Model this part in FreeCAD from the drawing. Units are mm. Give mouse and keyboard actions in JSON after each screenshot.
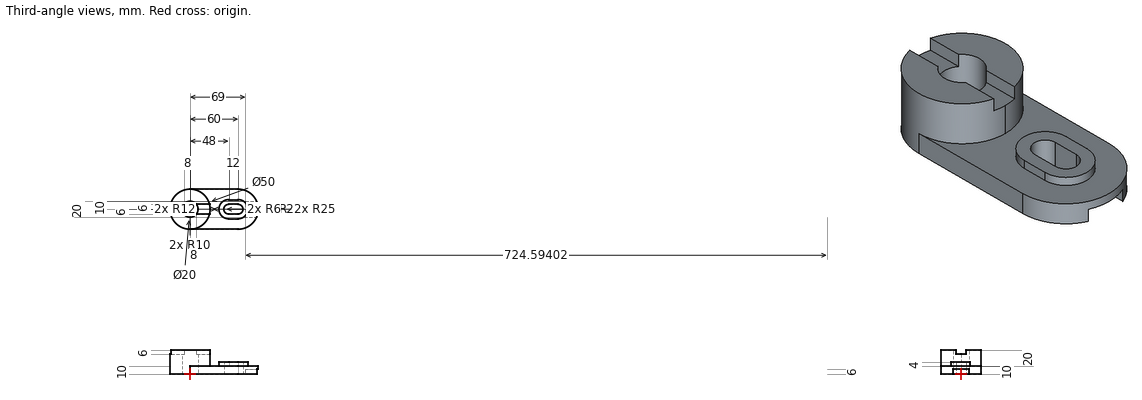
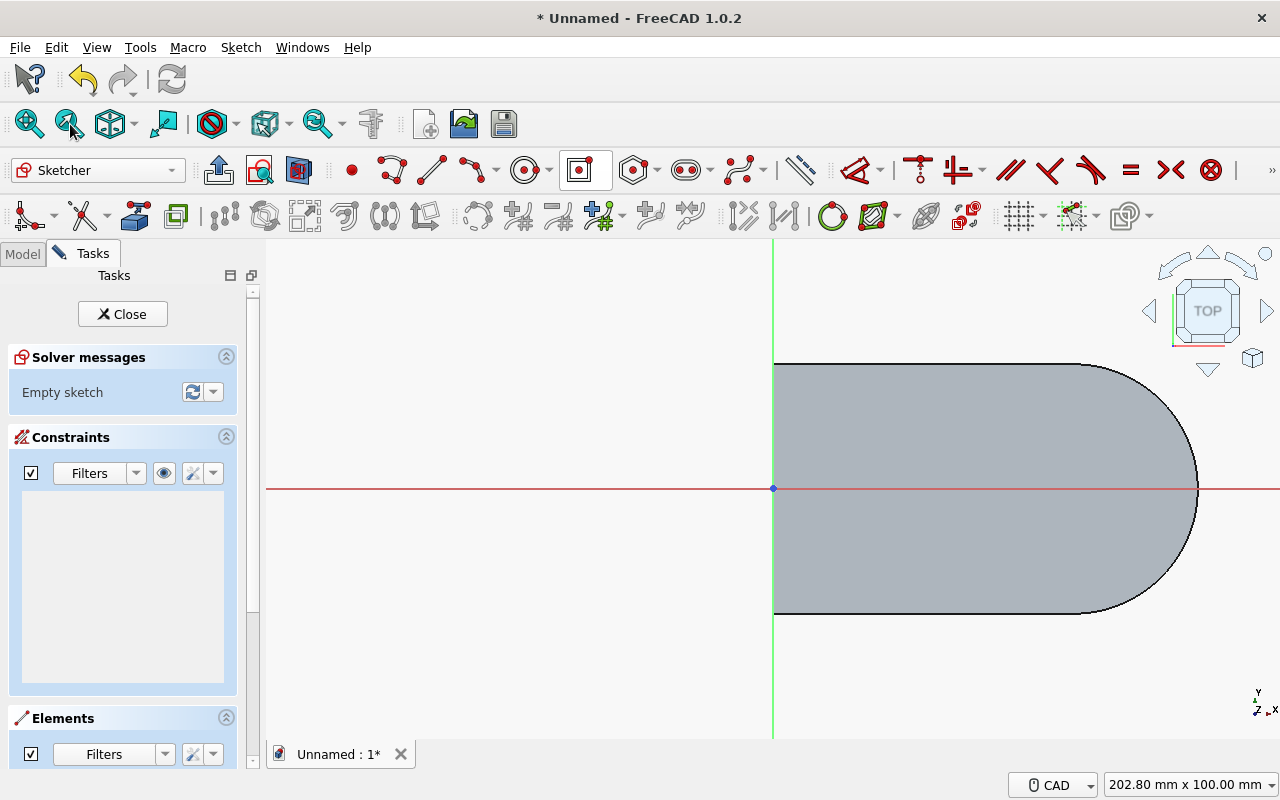
{"action": "left_click", "coordinate": [526, 170]}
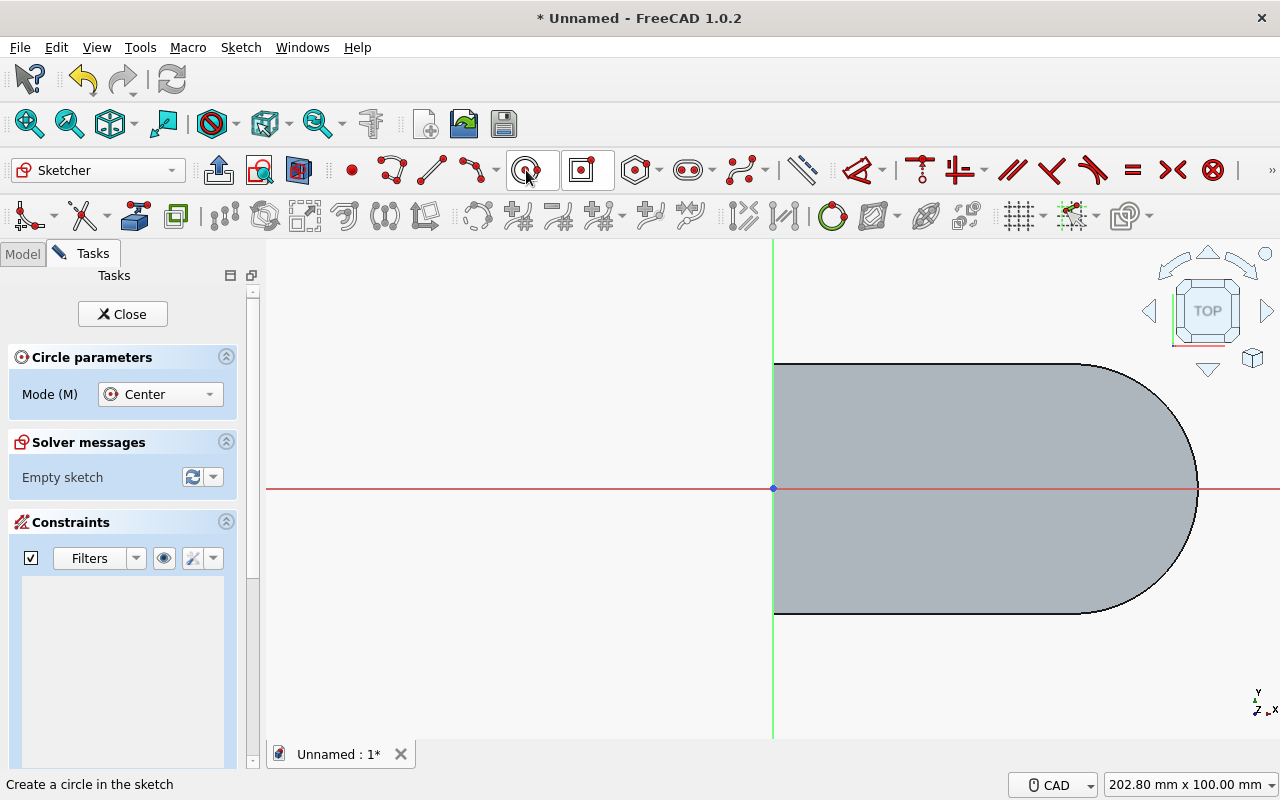
{"action": "left_click", "coordinate": [773, 489]}
{"action": "left_click", "coordinate": [861, 401]}
{"action": "key", "text": "Escape"}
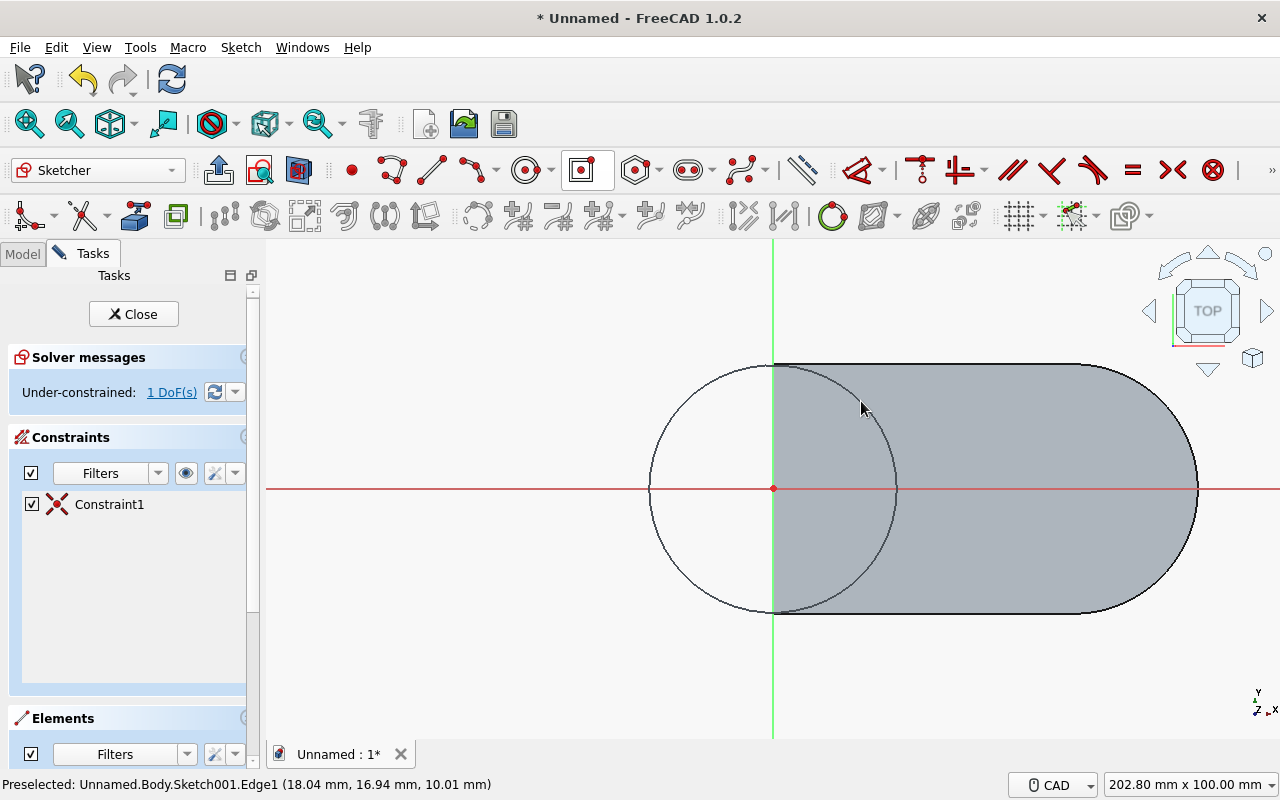
{"action": "left_click", "coordinate": [858, 170]}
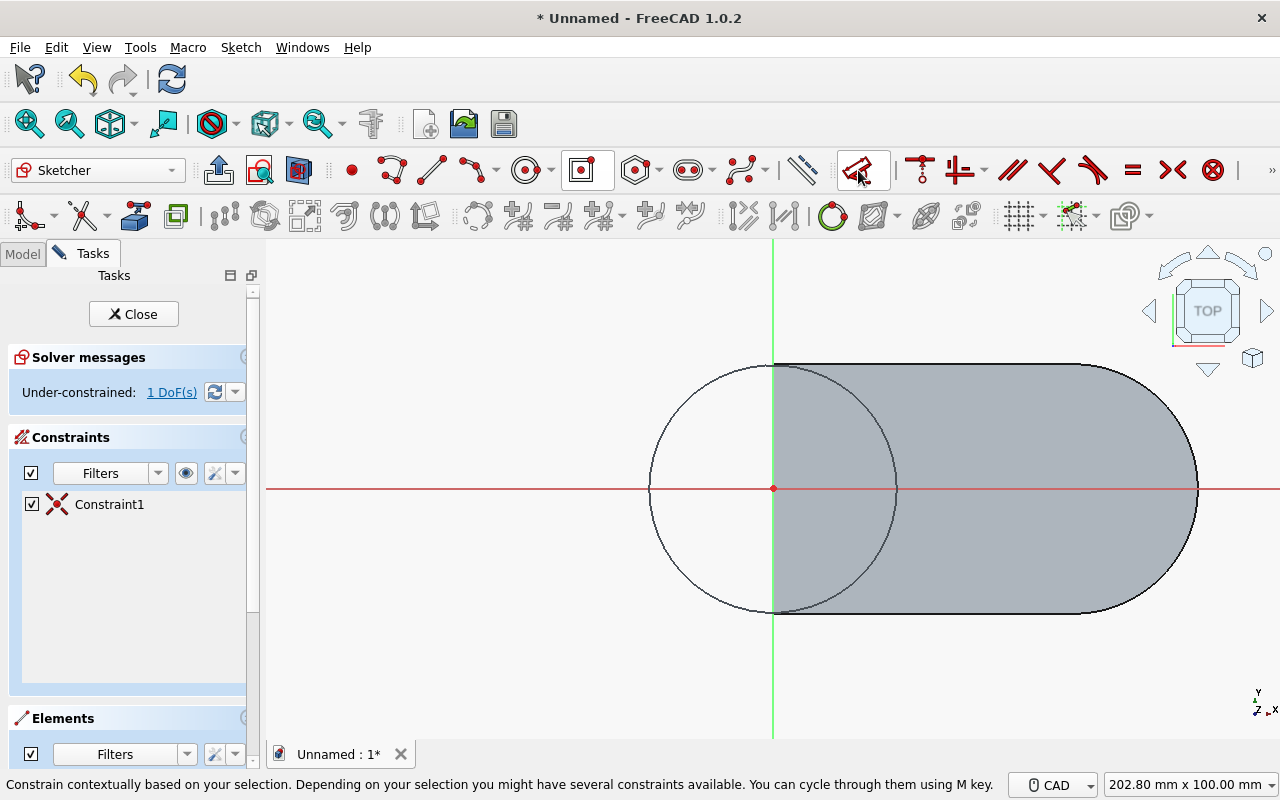
{"action": "left_click", "coordinate": [860, 401]}
{"action": "left_click", "coordinate": [882, 378]}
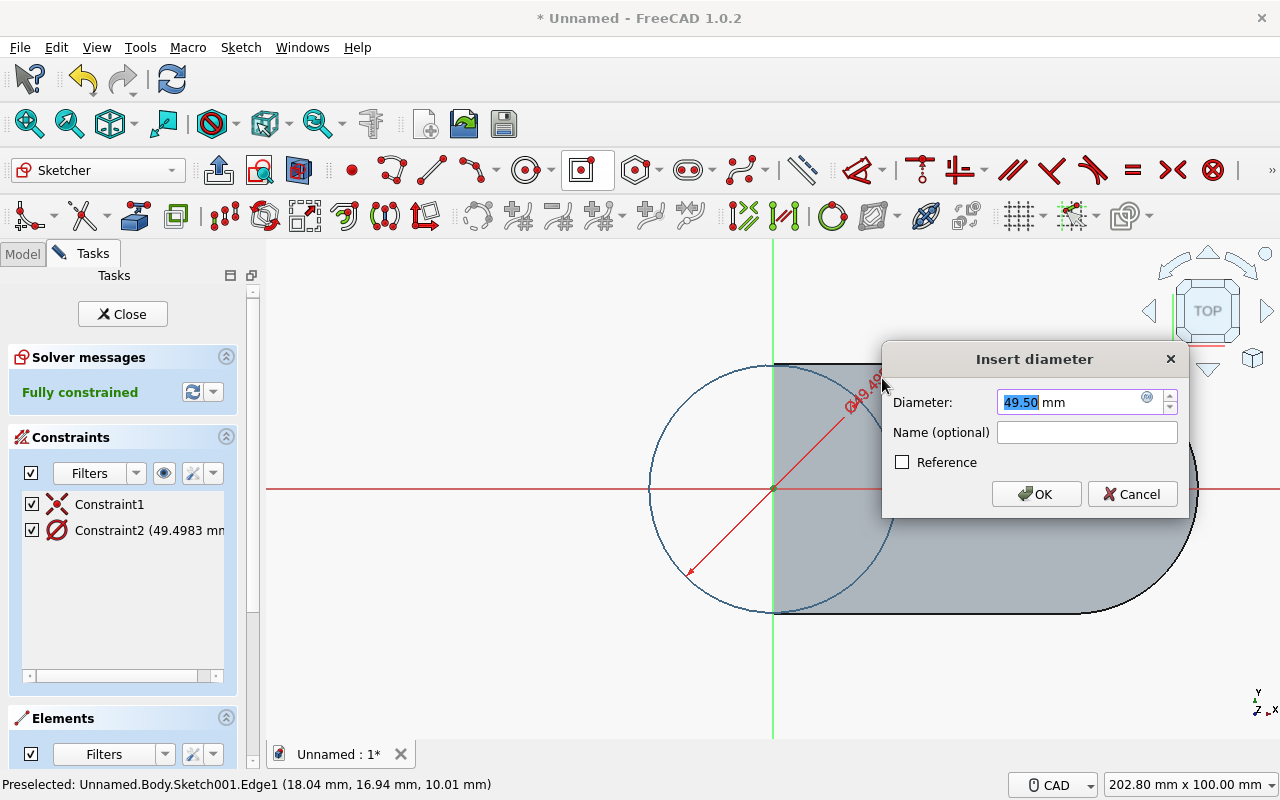
{"action": "type", "text": "50"}
{"action": "key", "text": "Return"}
{"action": "key", "text": "Escape"}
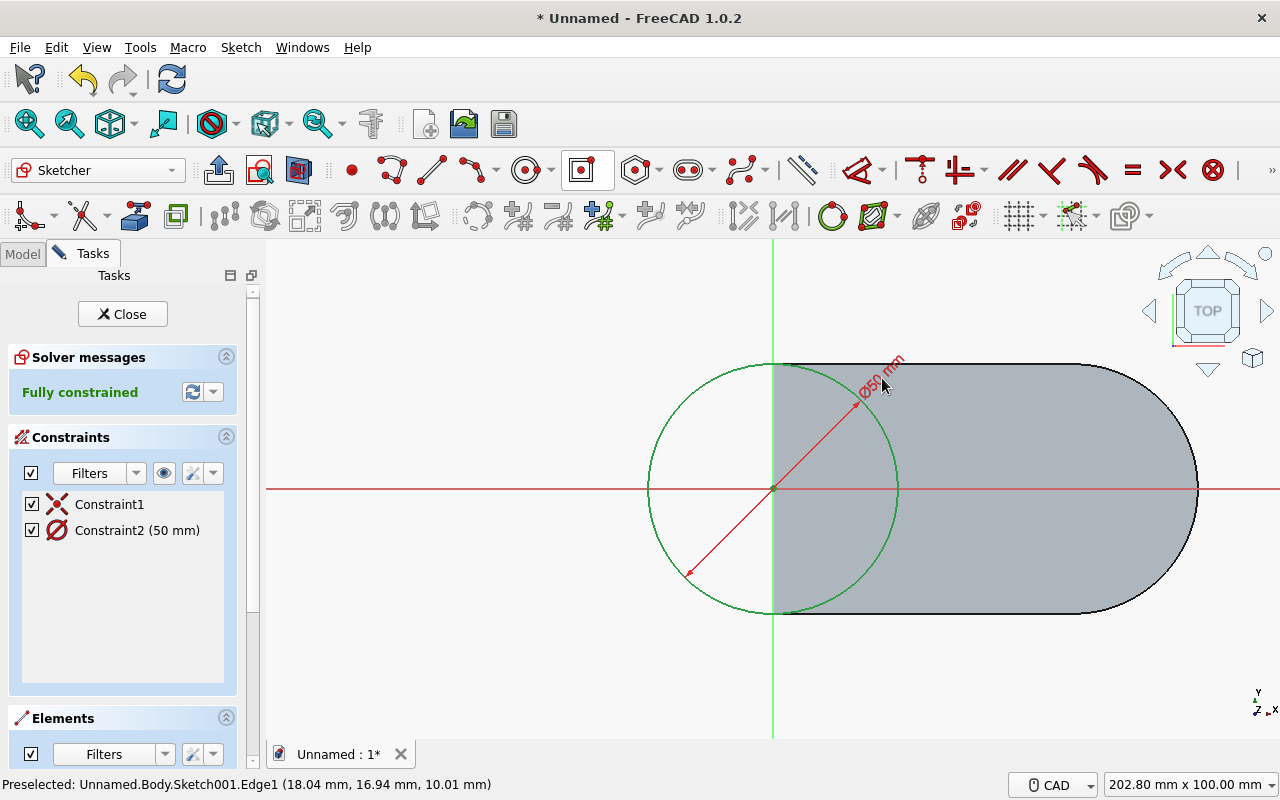
{"action": "left_click", "coordinate": [123, 314]}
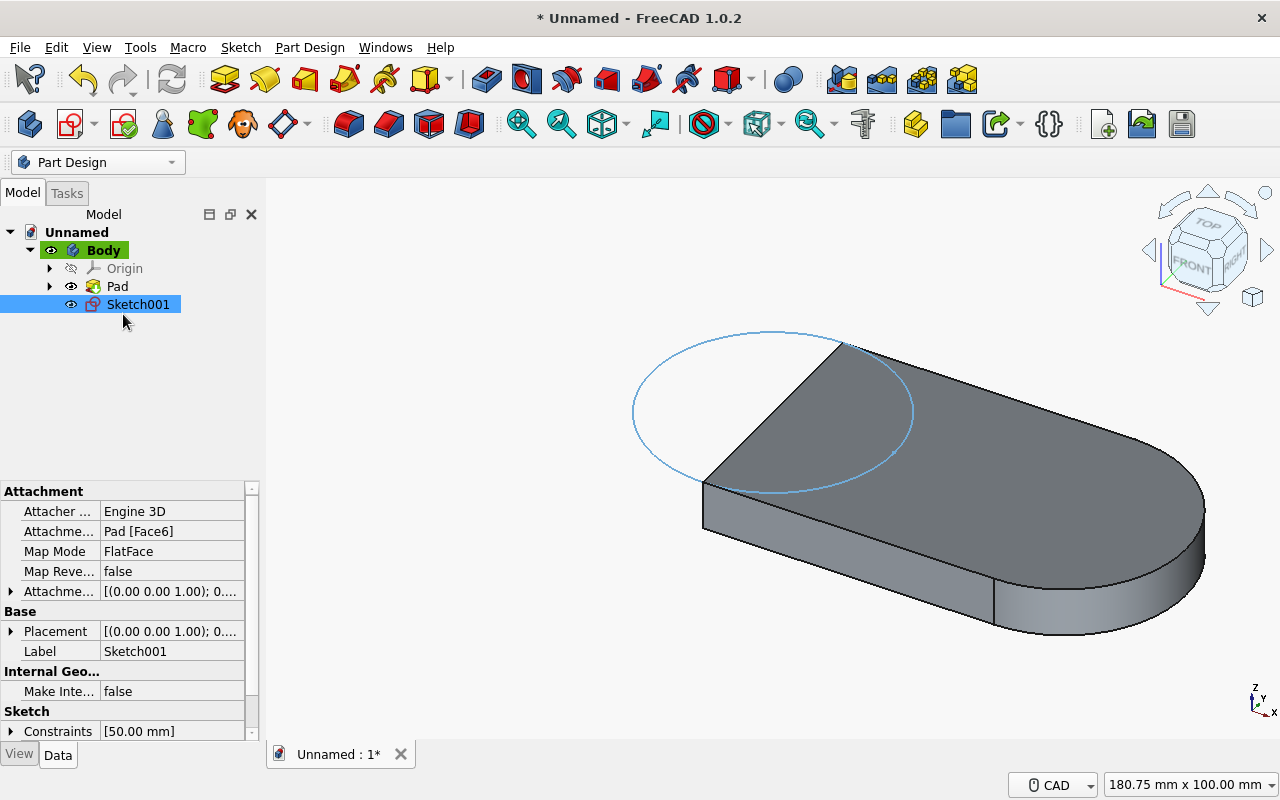
{"action": "left_click", "coordinate": [226, 80]}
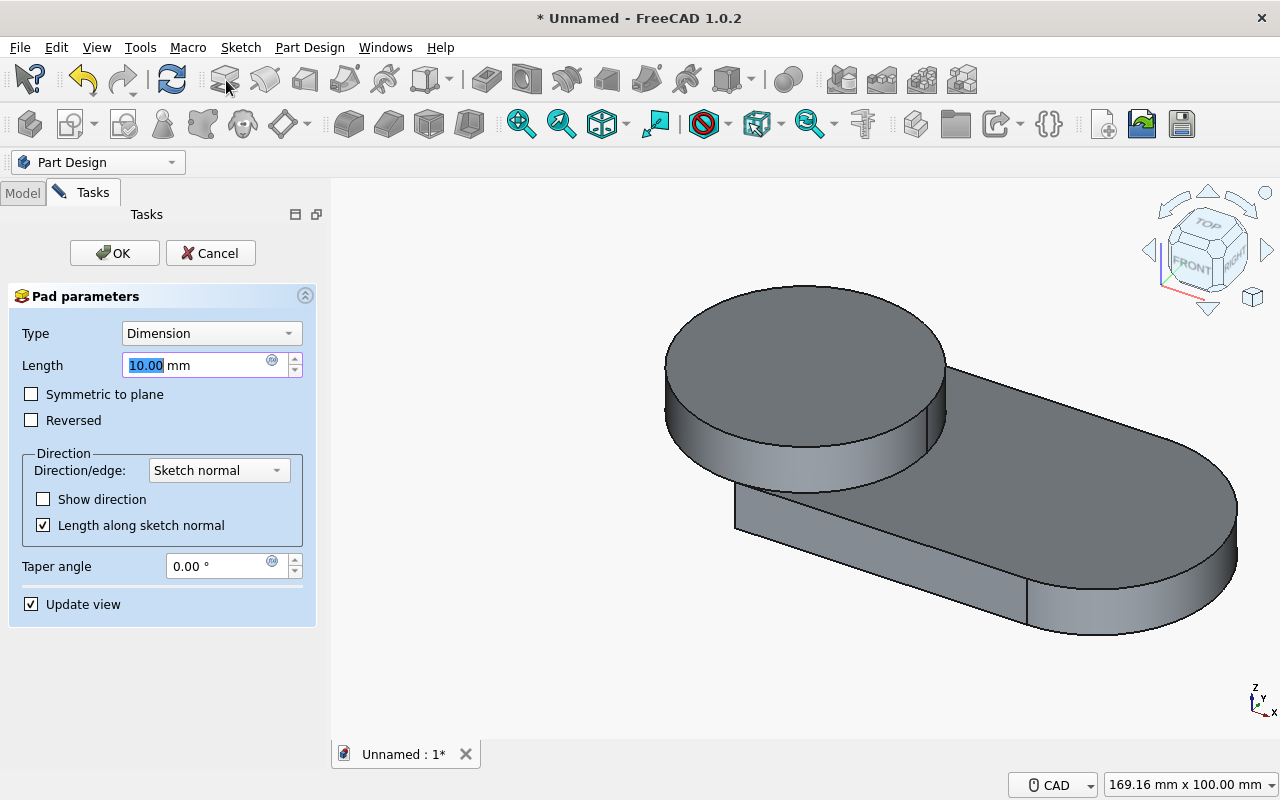
{"action": "type", "text": "10"}
{"action": "key", "text": "Tab"}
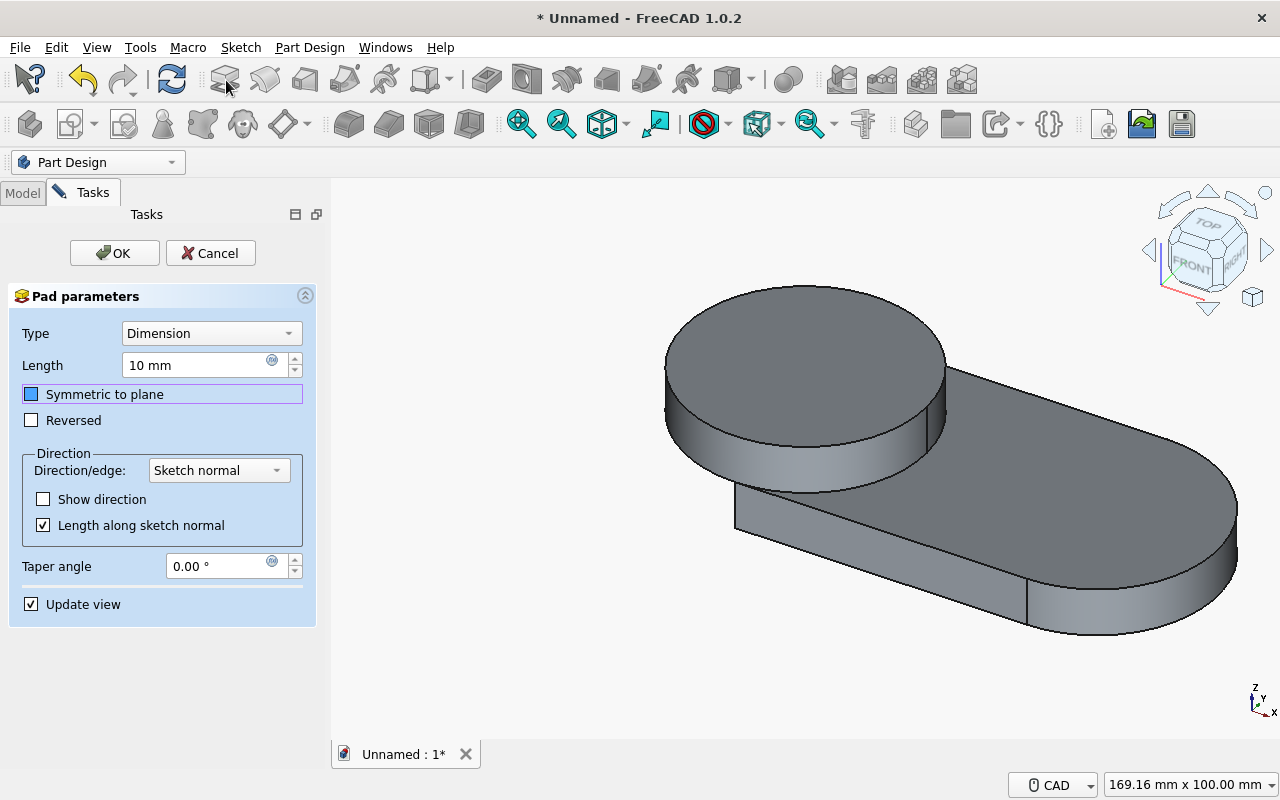
{"action": "left_click", "coordinate": [30, 420]}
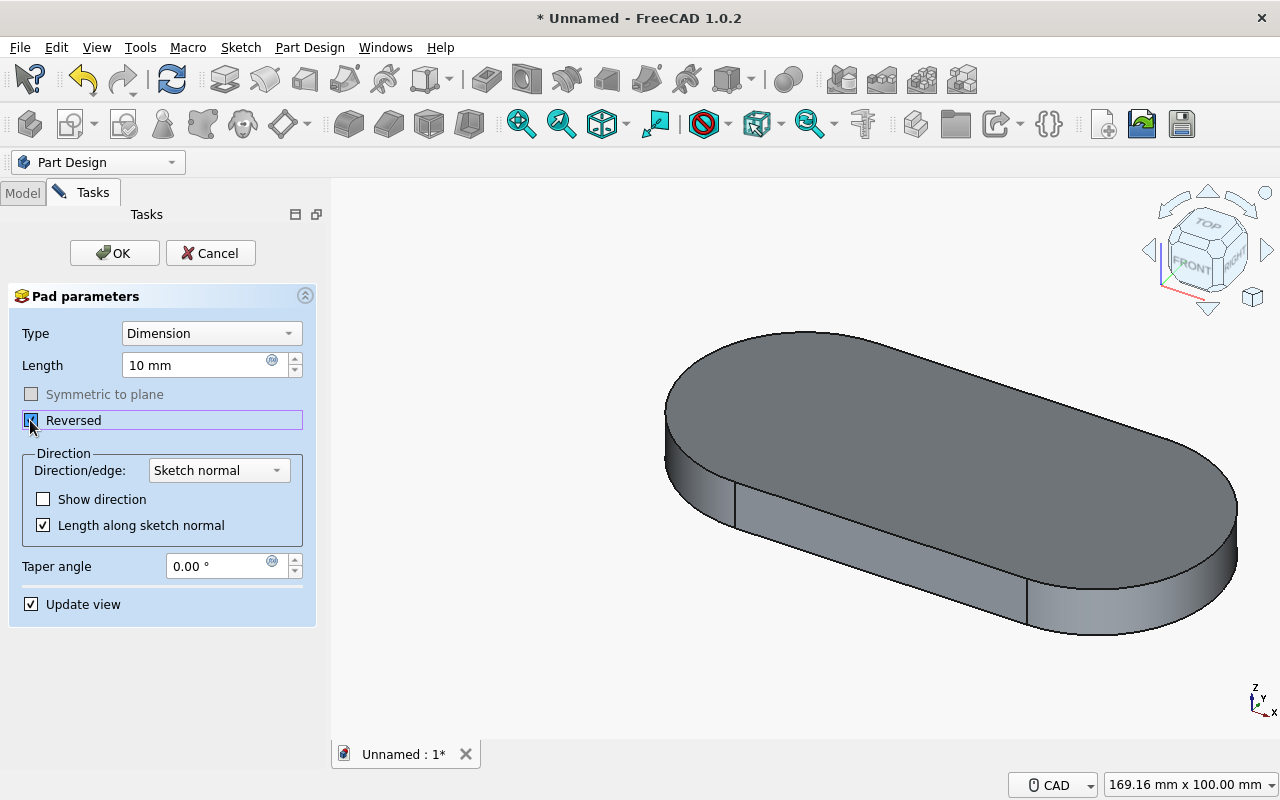
{"action": "left_click", "coordinate": [115, 253]}